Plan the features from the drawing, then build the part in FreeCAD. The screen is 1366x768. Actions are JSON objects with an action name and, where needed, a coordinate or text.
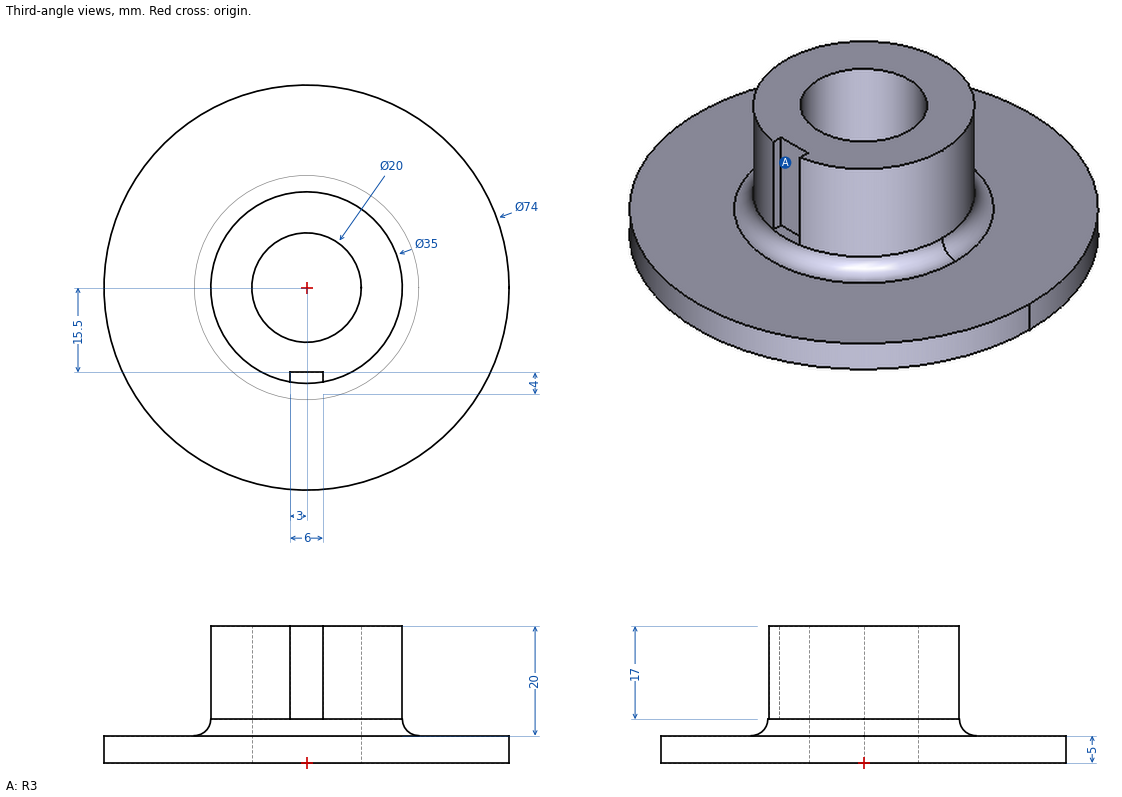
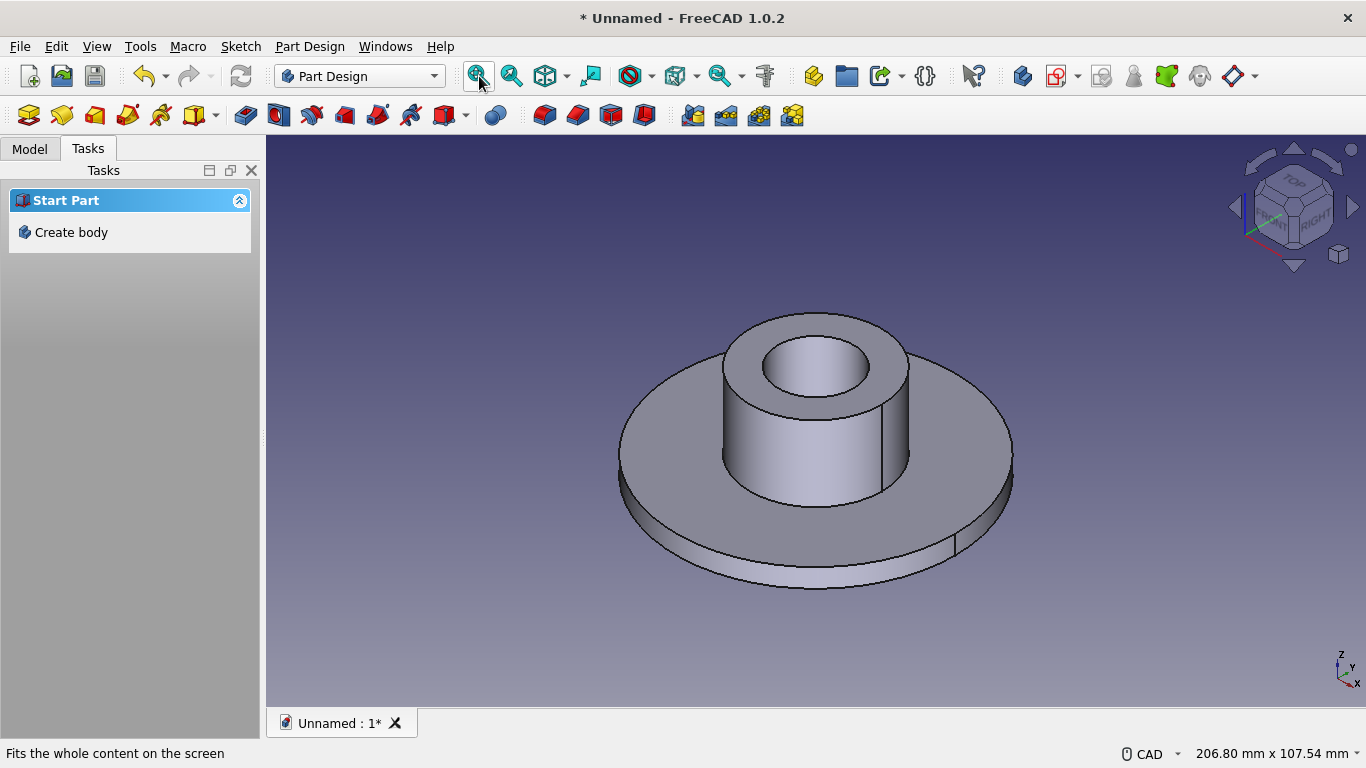
{"action": "key", "text": "2"}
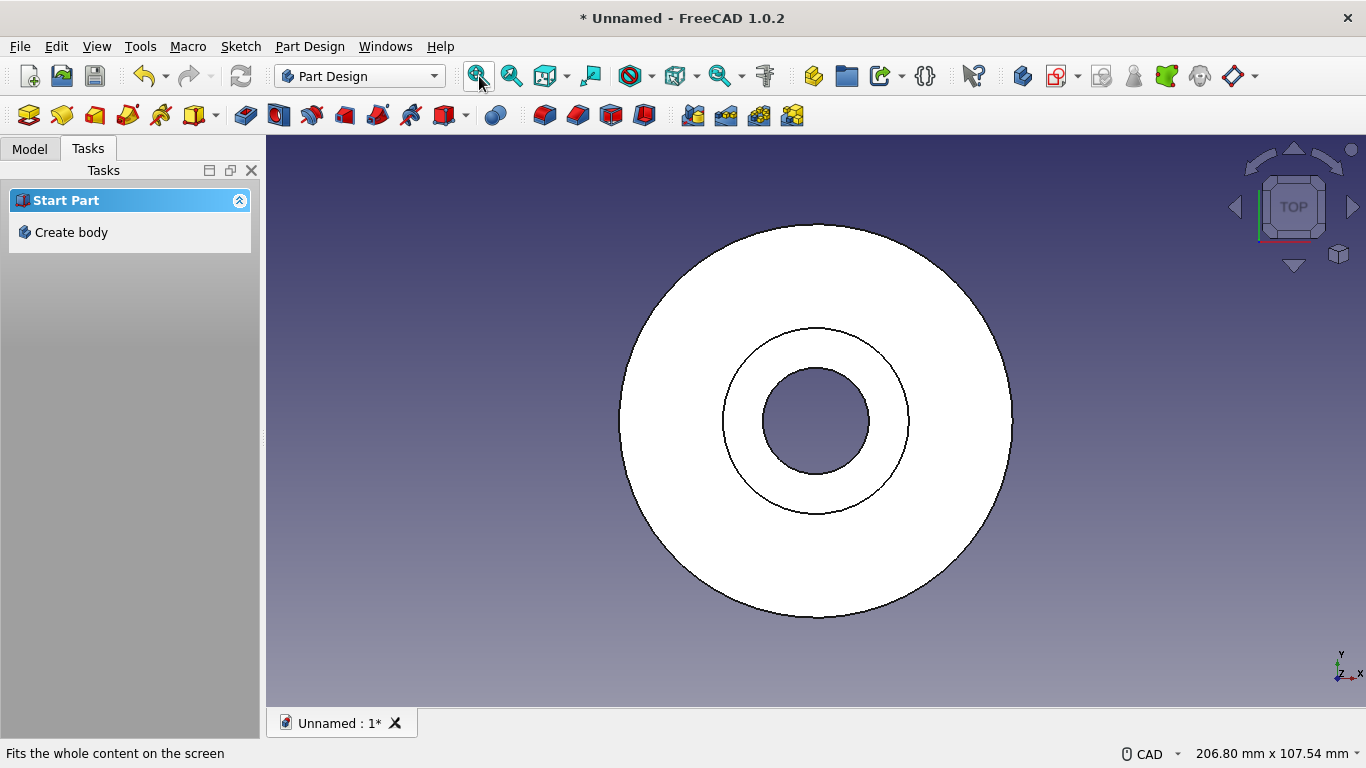
{"action": "key", "text": "1"}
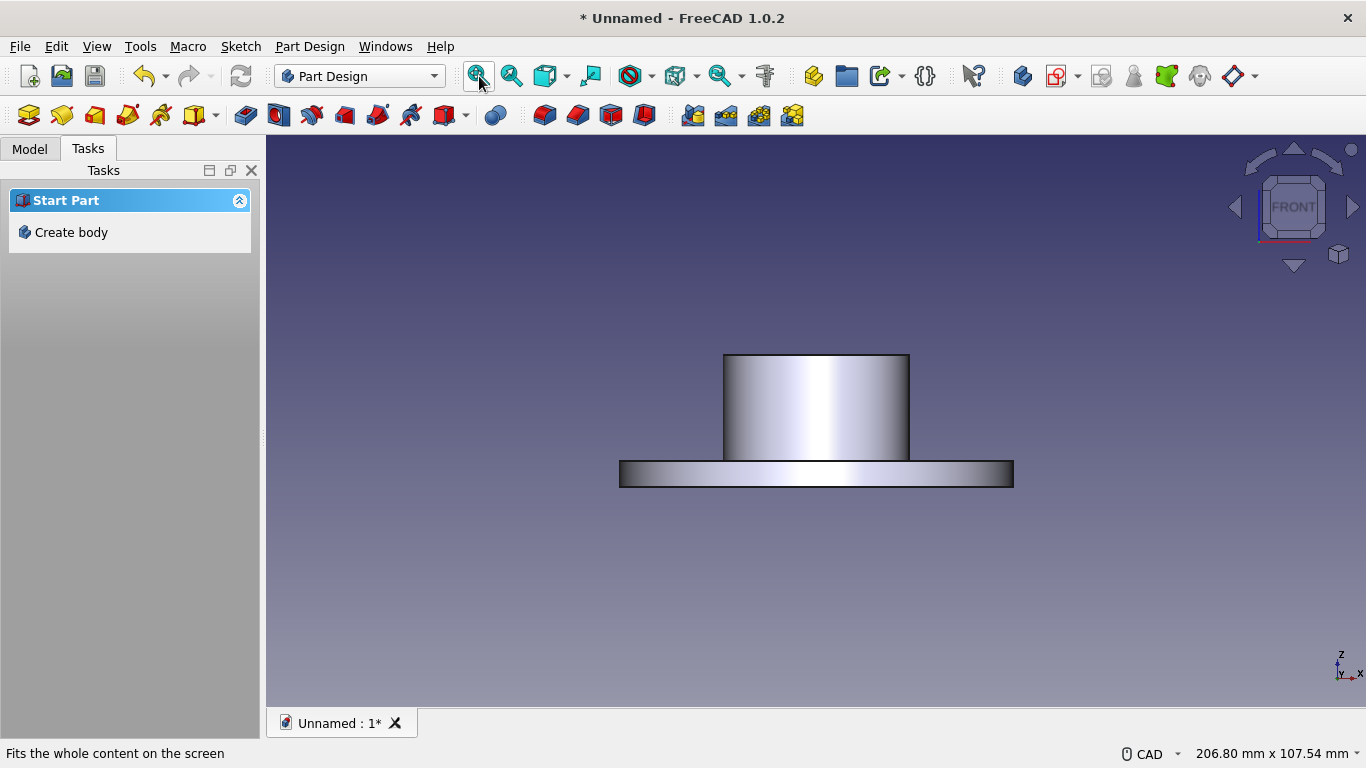
{"action": "left_click", "coordinate": [479, 76]}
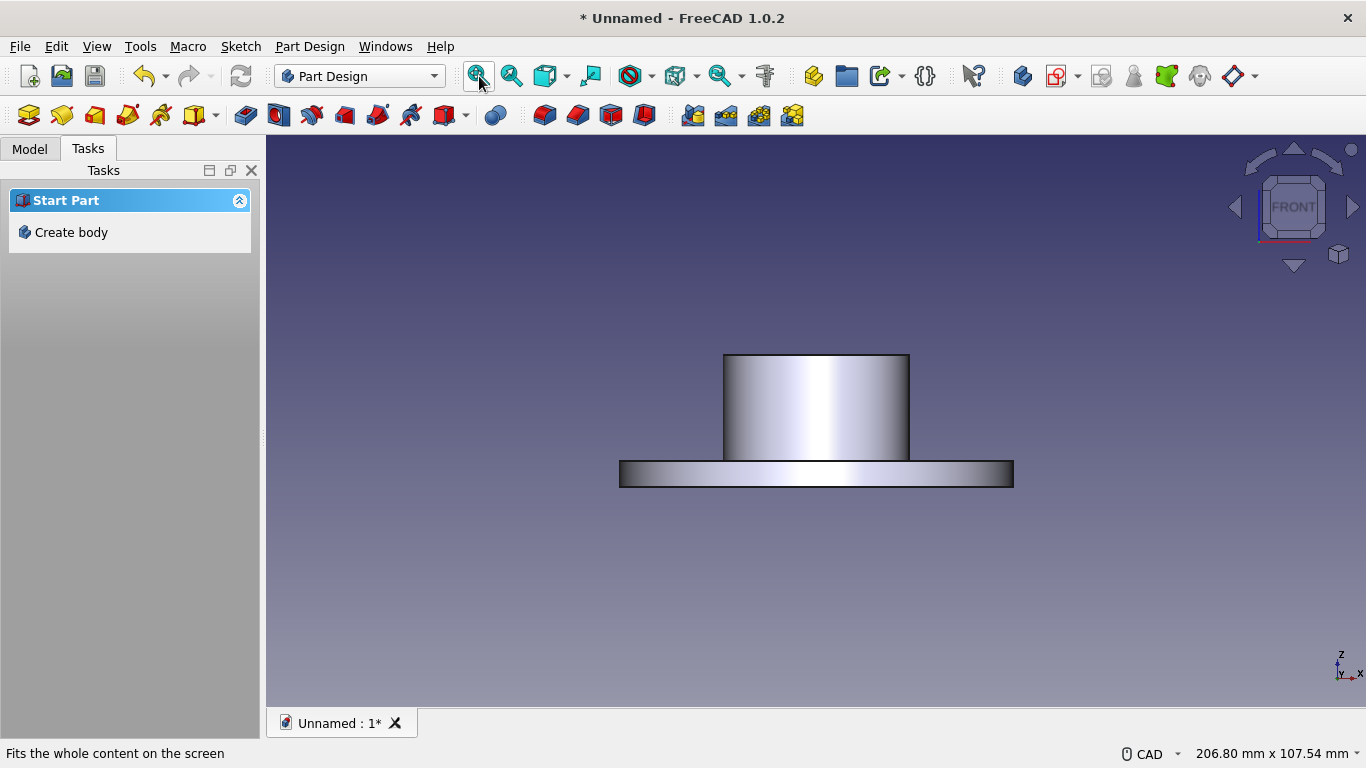
{"action": "key", "text": "3"}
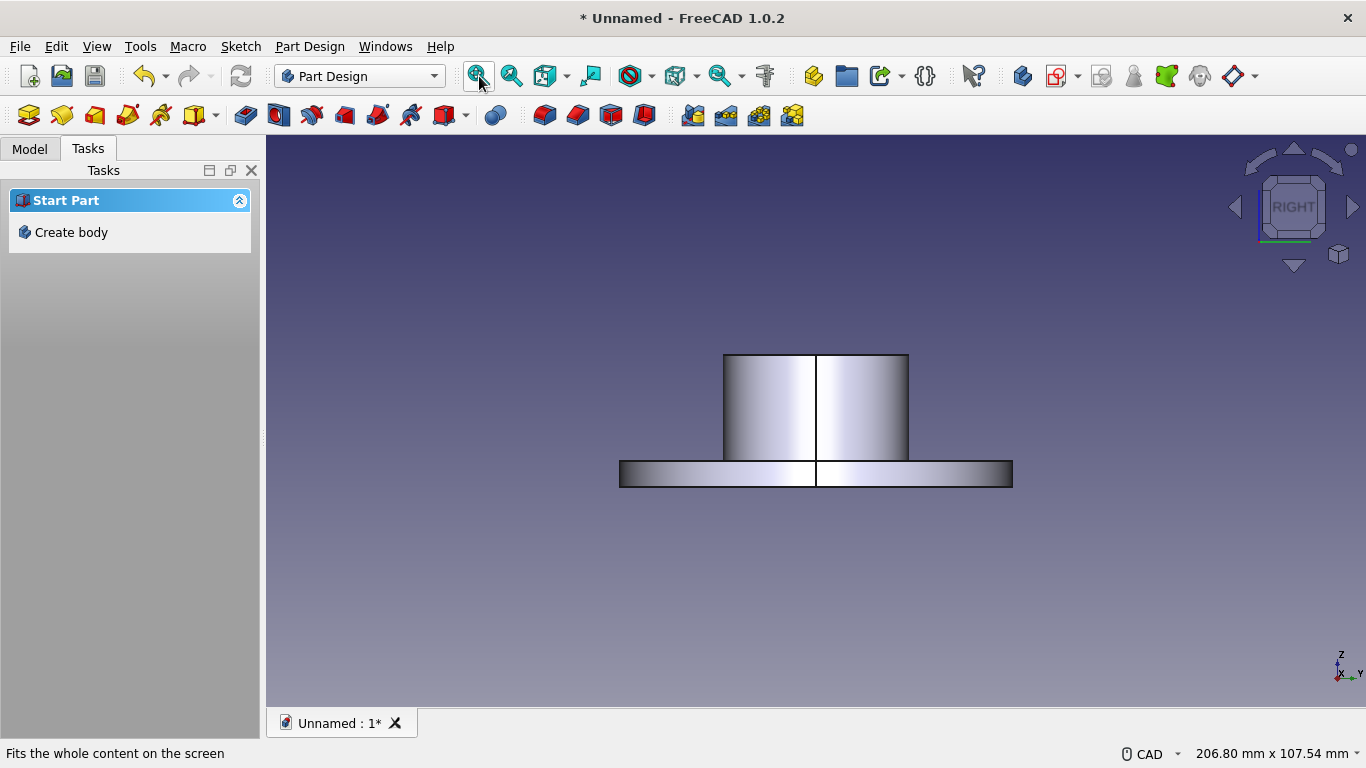
{"action": "left_click", "coordinate": [479, 76]}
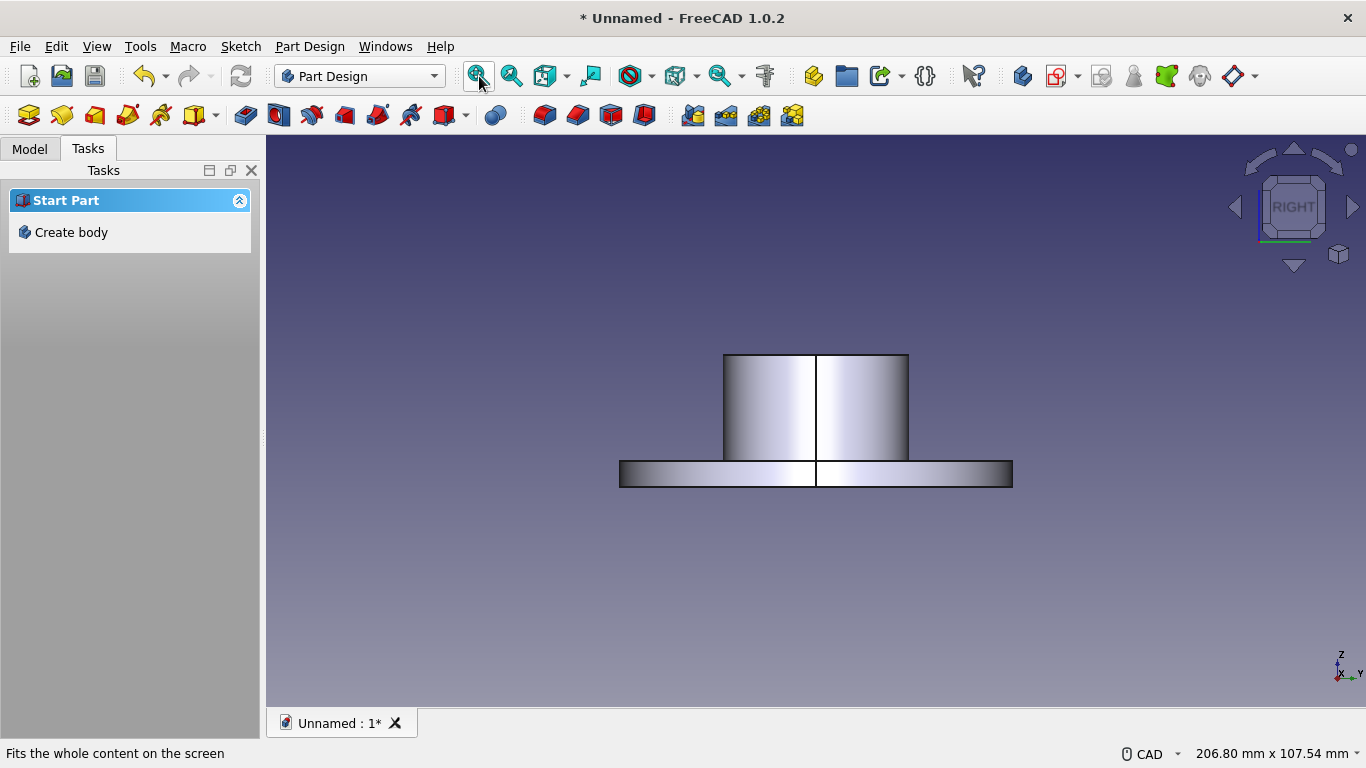
{"action": "key", "text": "5"}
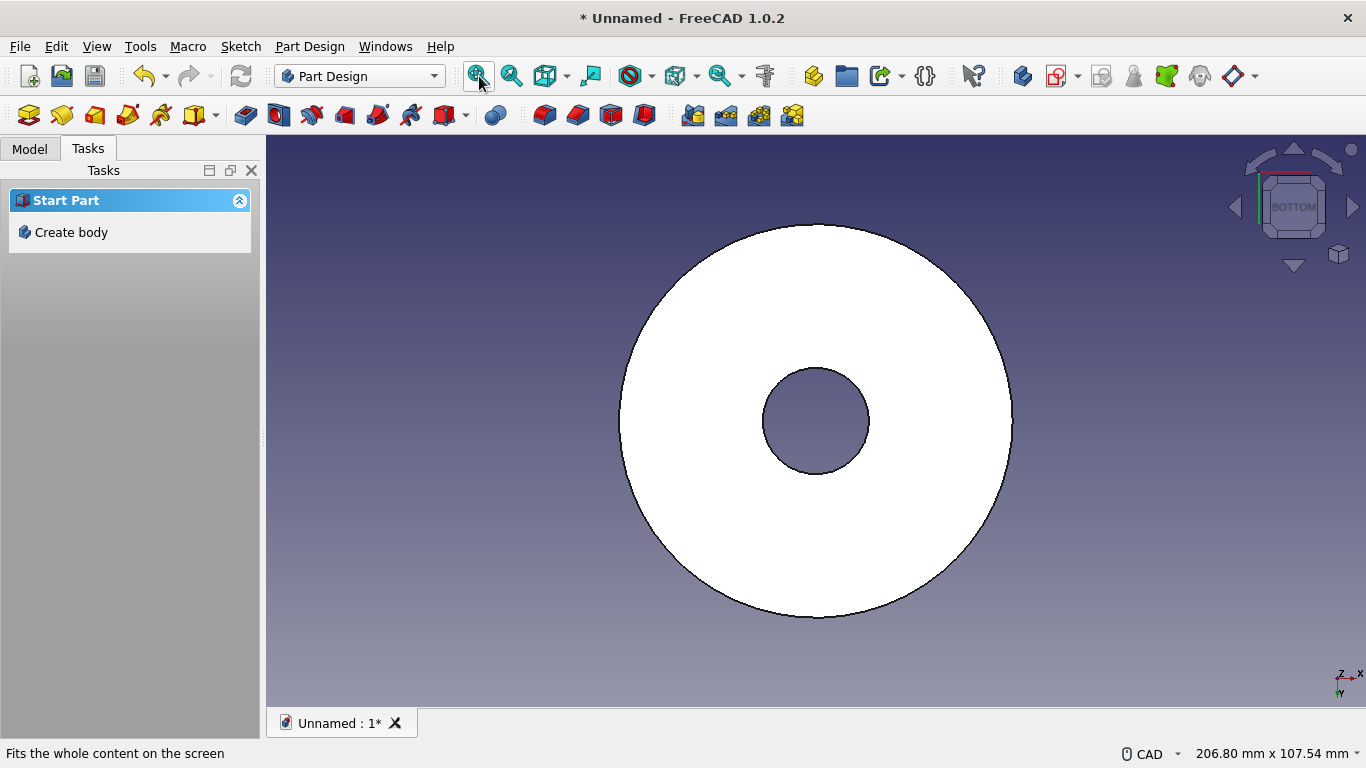
{"action": "key", "text": "4"}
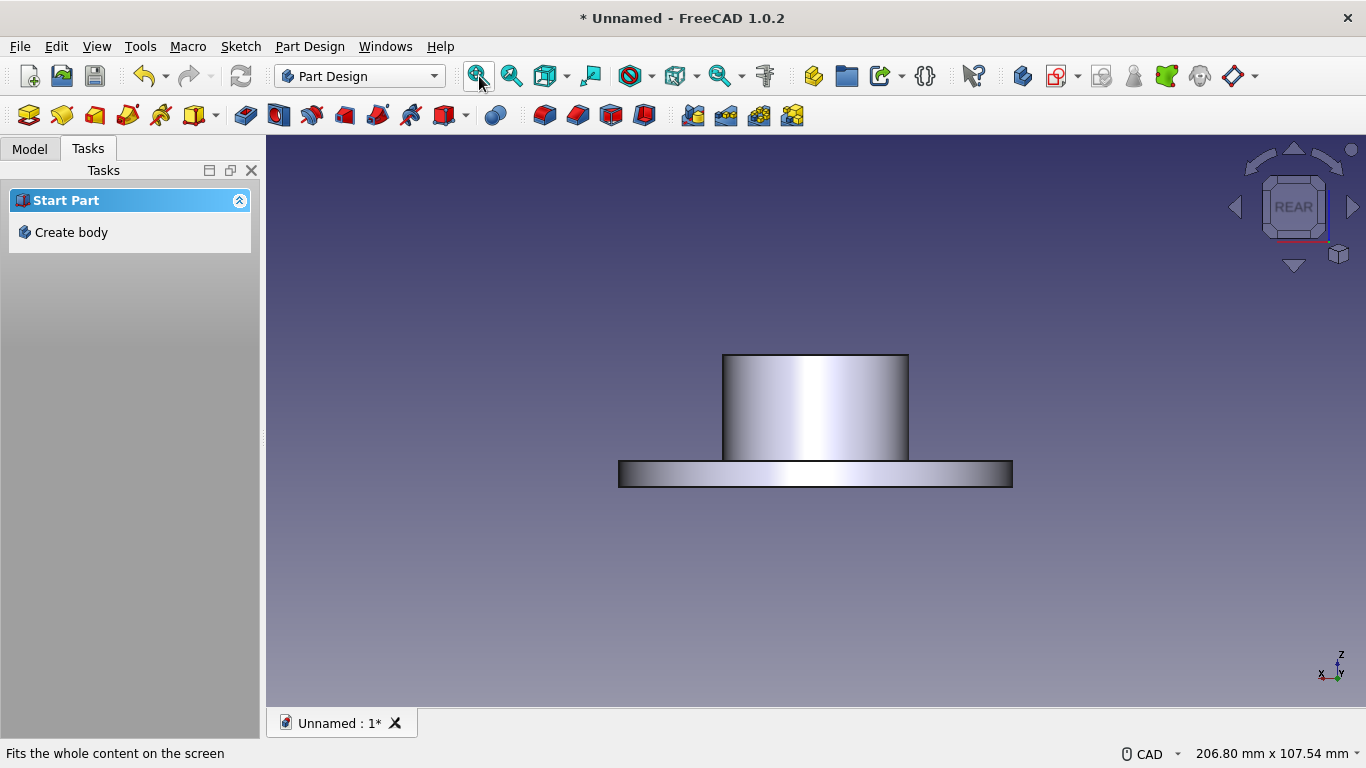
{"action": "left_click", "coordinate": [479, 76]}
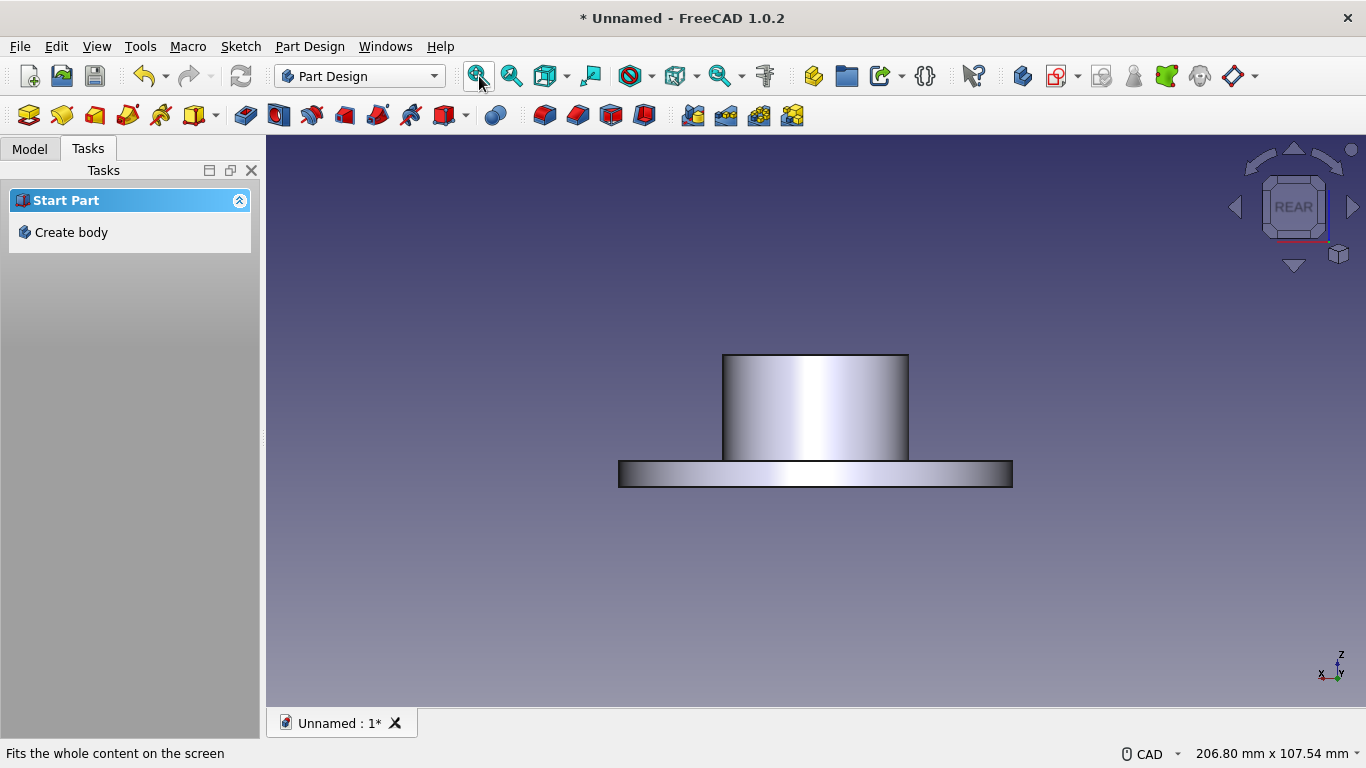
{"action": "key", "text": "6"}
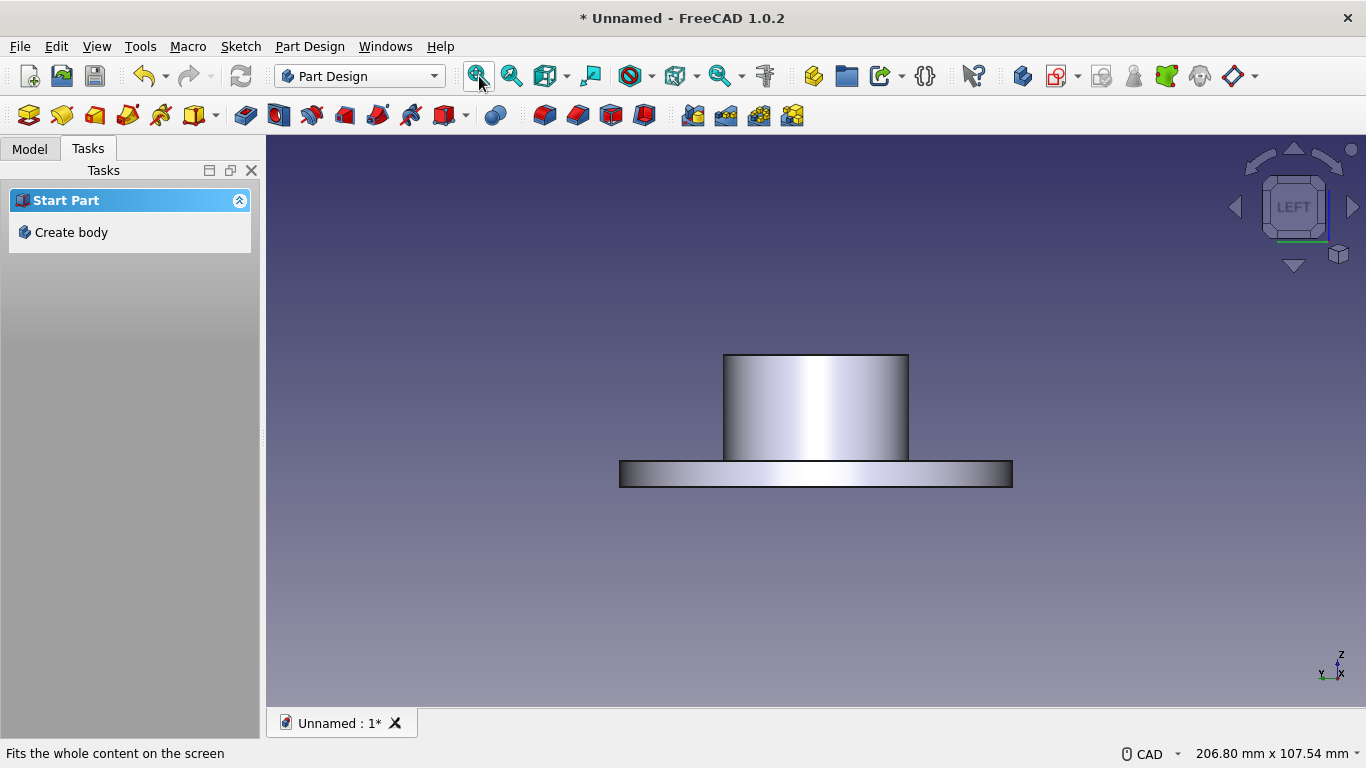
{"action": "left_click", "coordinate": [479, 76]}